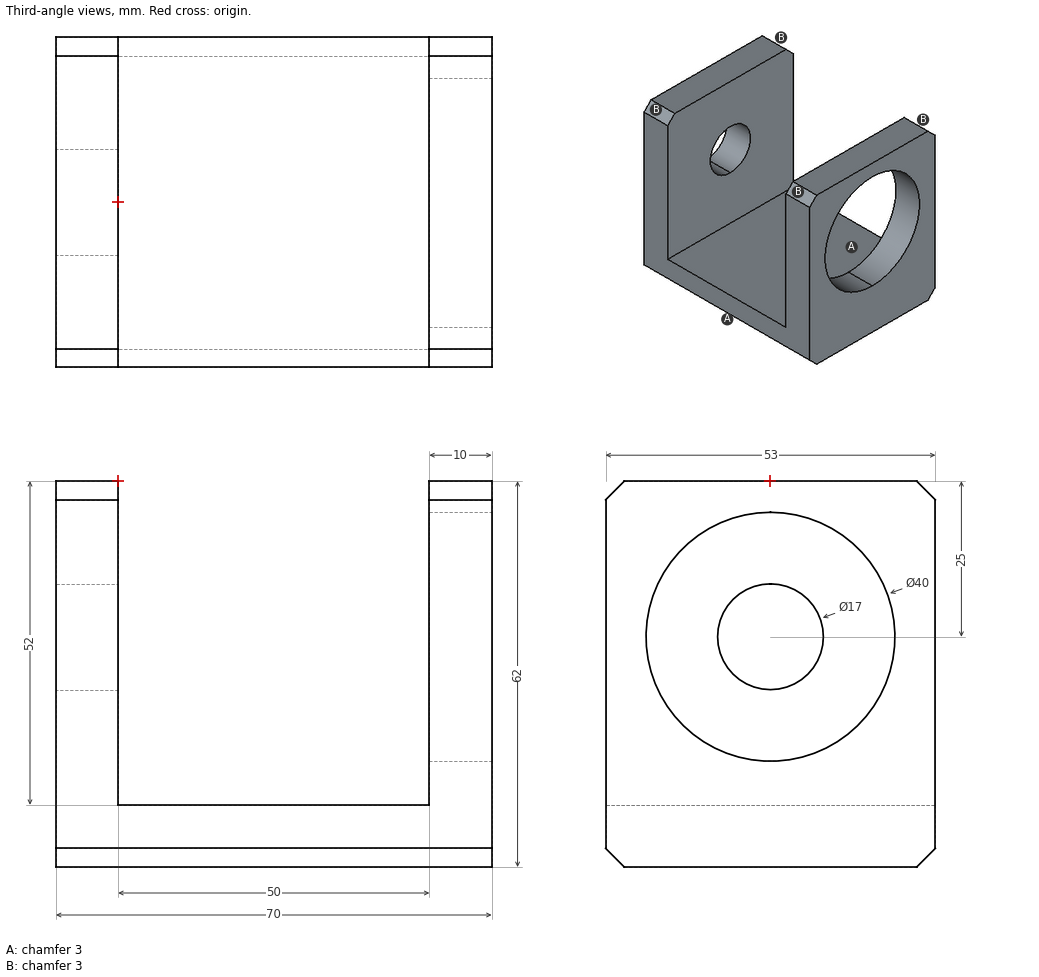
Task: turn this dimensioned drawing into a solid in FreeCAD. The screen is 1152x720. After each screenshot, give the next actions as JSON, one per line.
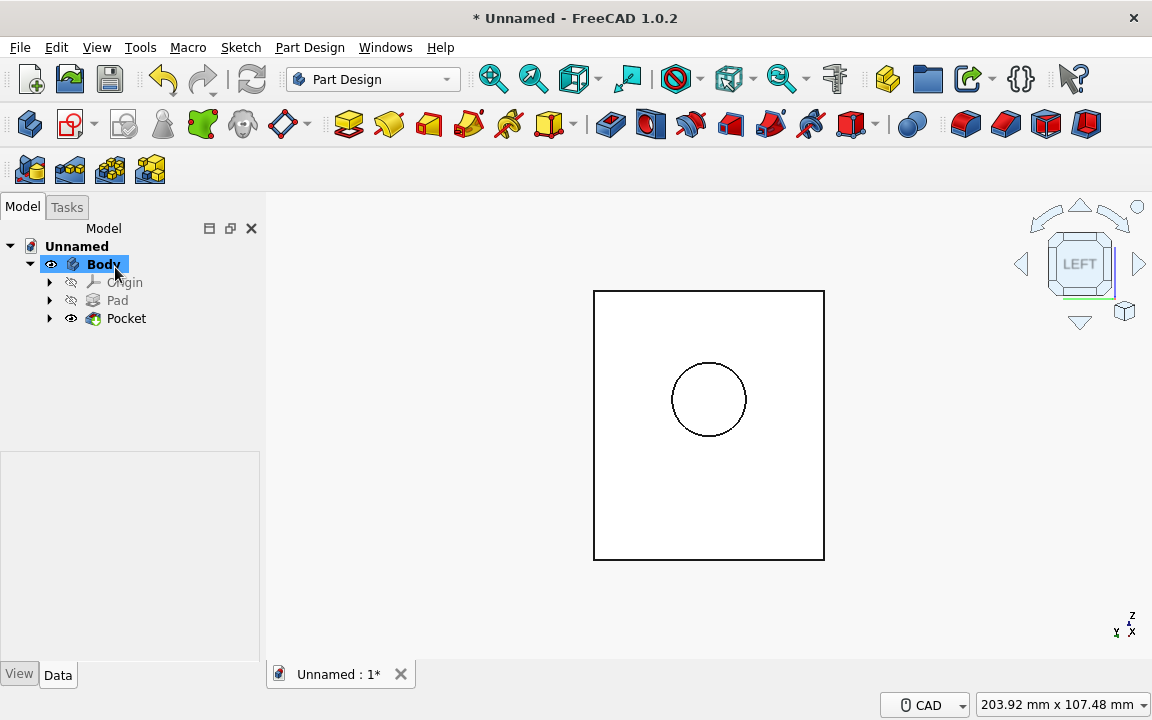
{"action": "left_click", "coordinate": [709, 403]}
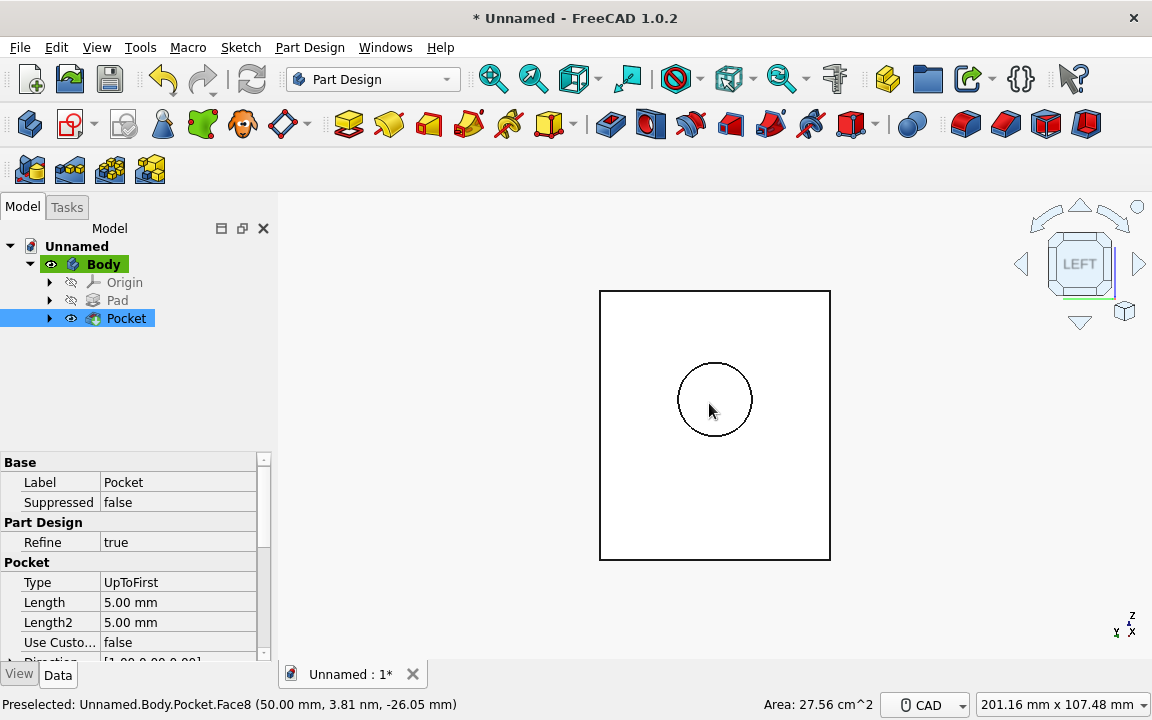
{"action": "left_click", "coordinate": [70, 124]}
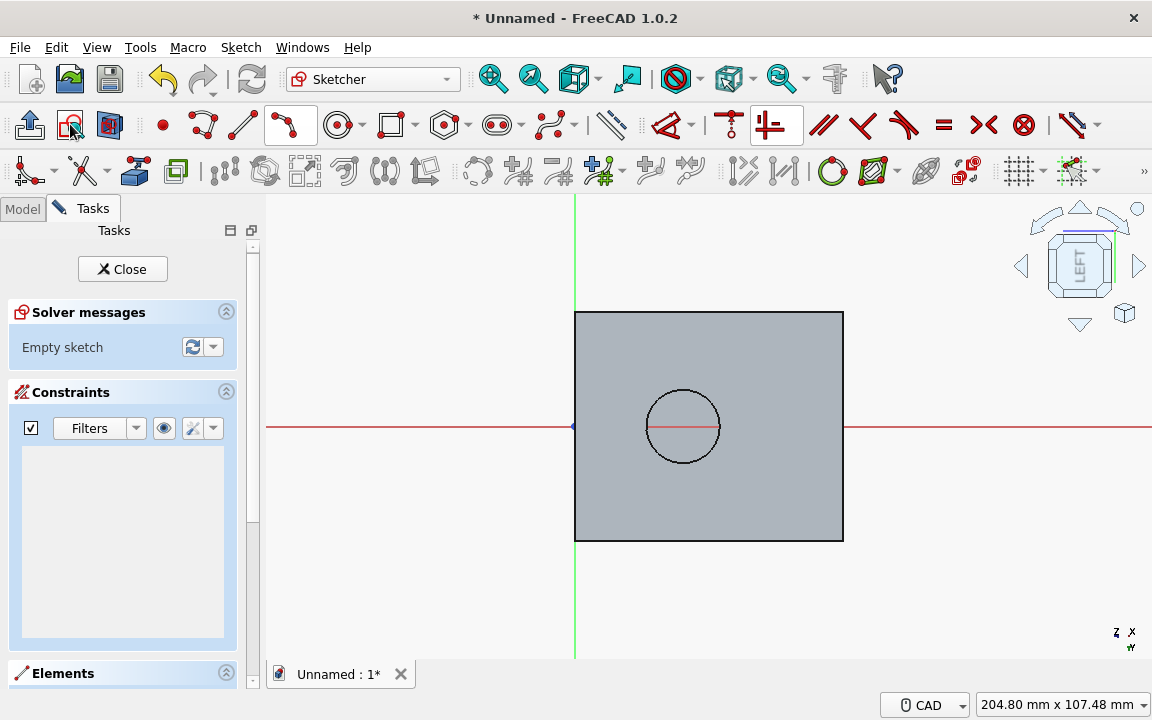
{"action": "left_click", "coordinate": [110, 126]}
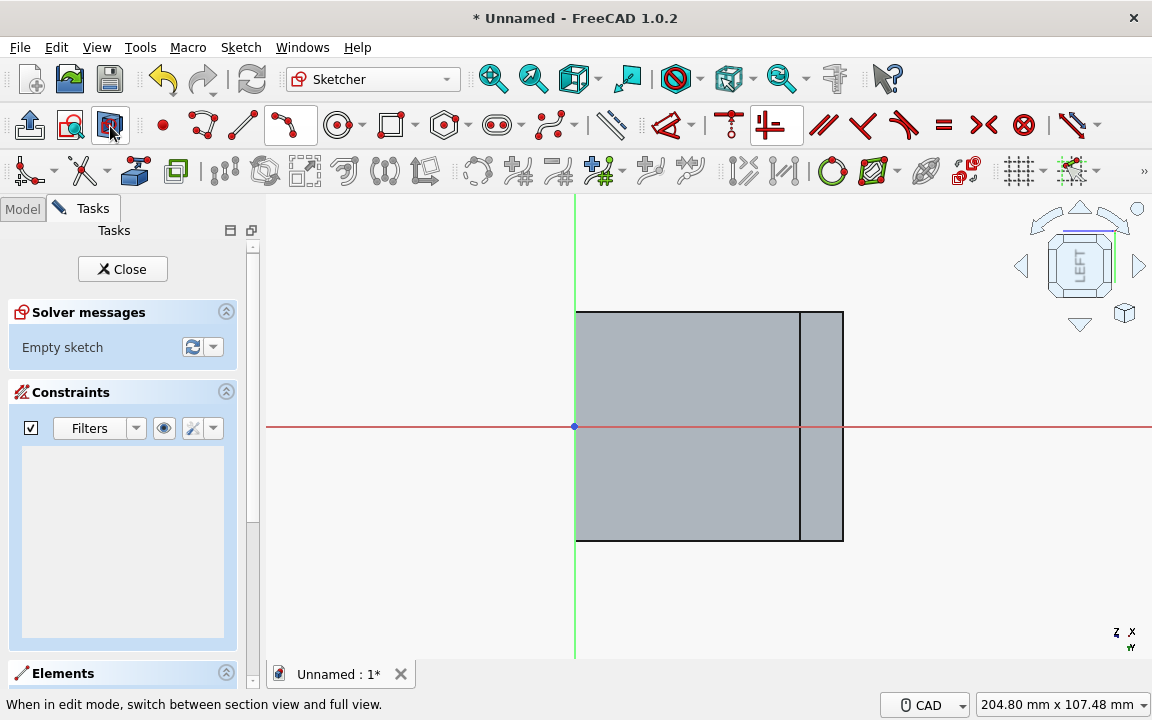
{"action": "scroll", "coordinate": [711, 426], "scroll_direction": "up", "scroll_amount": 3}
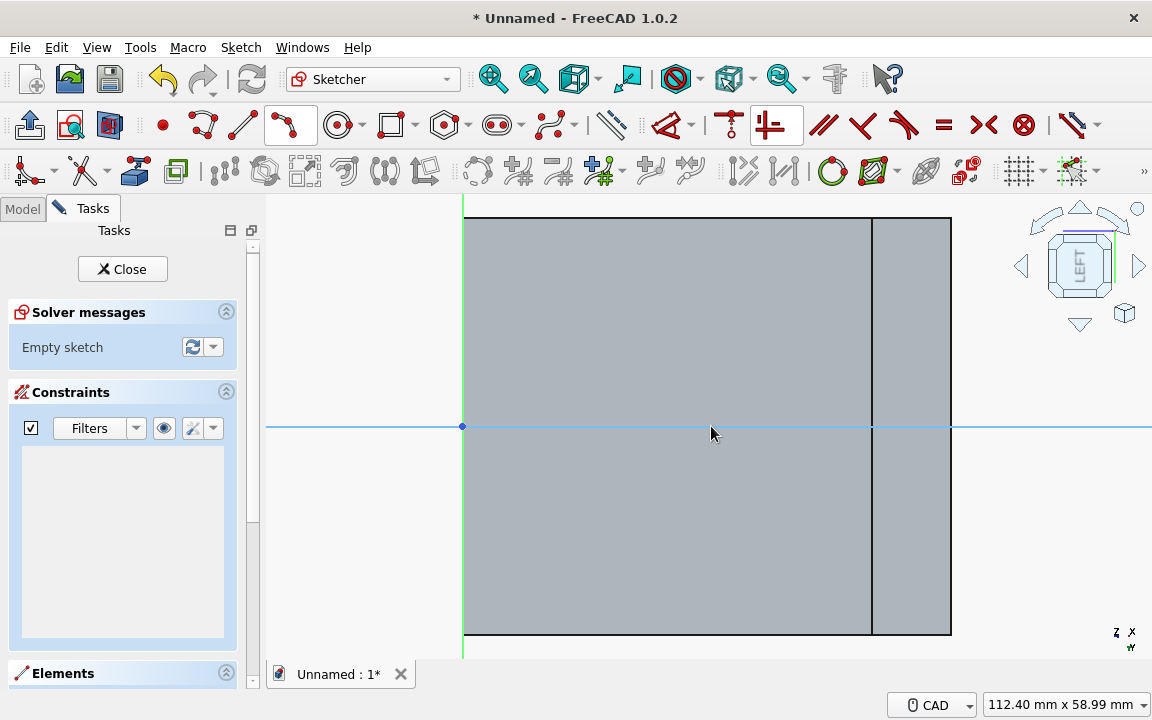
{"action": "key", "text": "g c"}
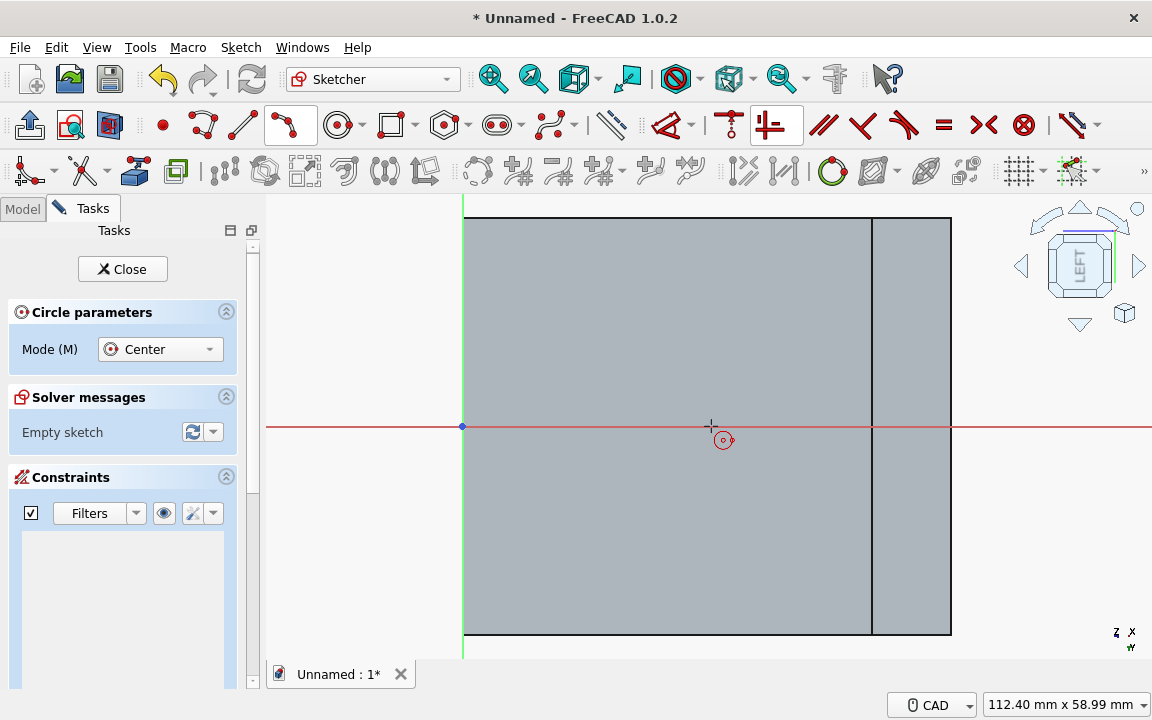
{"action": "left_click", "coordinate": [660, 426]}
{"action": "left_click", "coordinate": [771, 315]}
{"action": "key", "text": "Escape"}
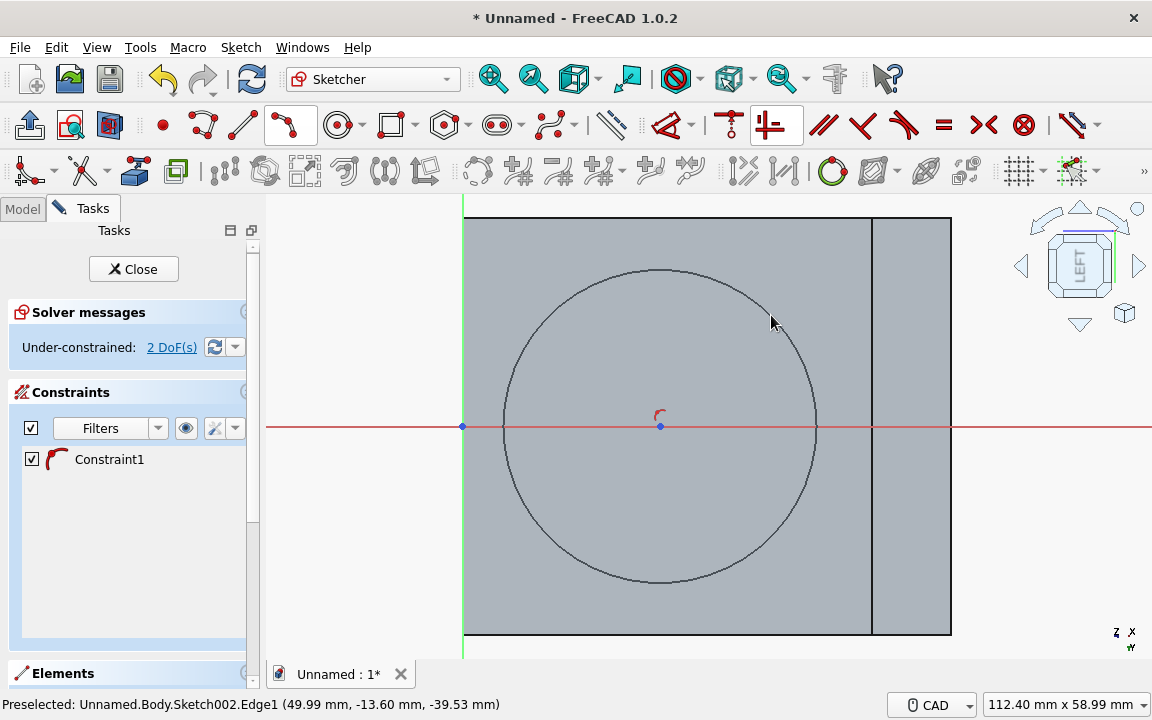
{"action": "key", "text": "d"}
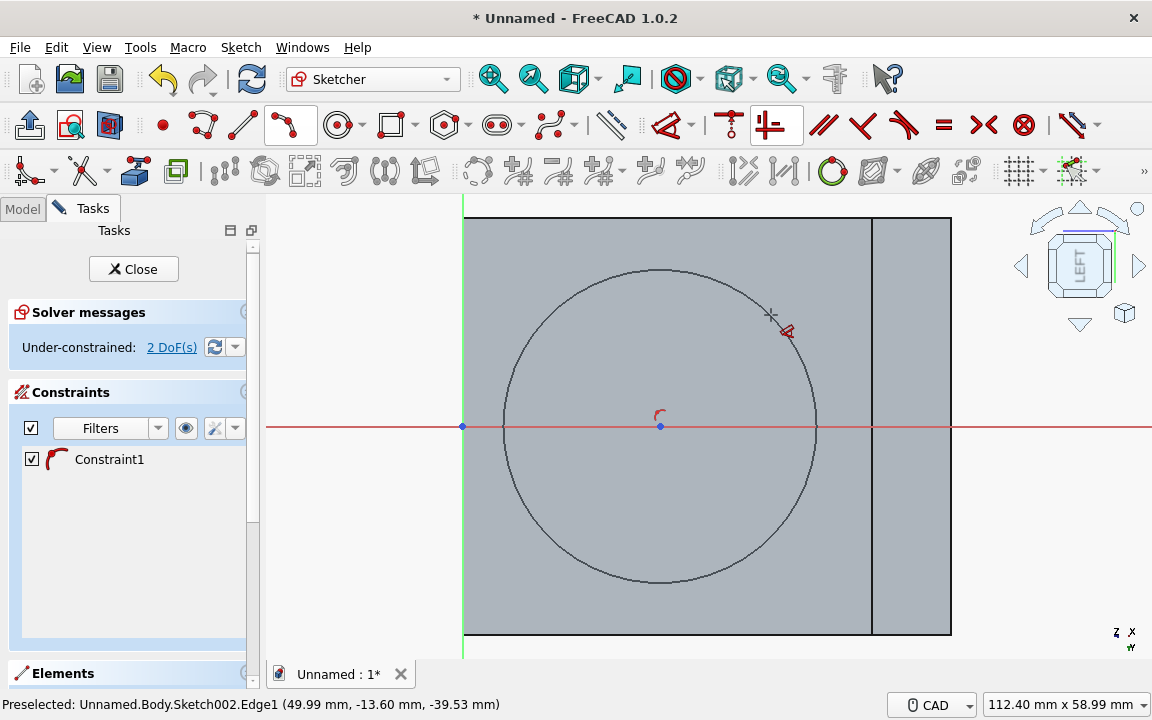
{"action": "left_click", "coordinate": [770, 315]}
{"action": "left_click", "coordinate": [792, 292]}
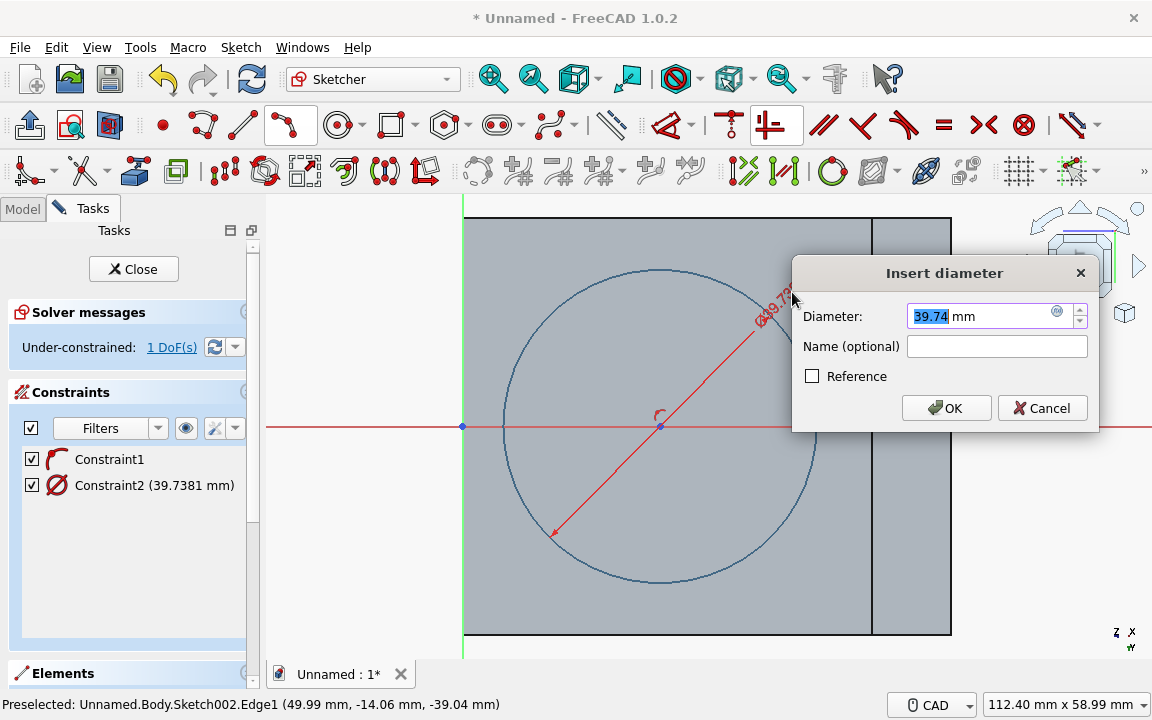
{"action": "type", "text": "40"}
{"action": "key", "text": "Return"}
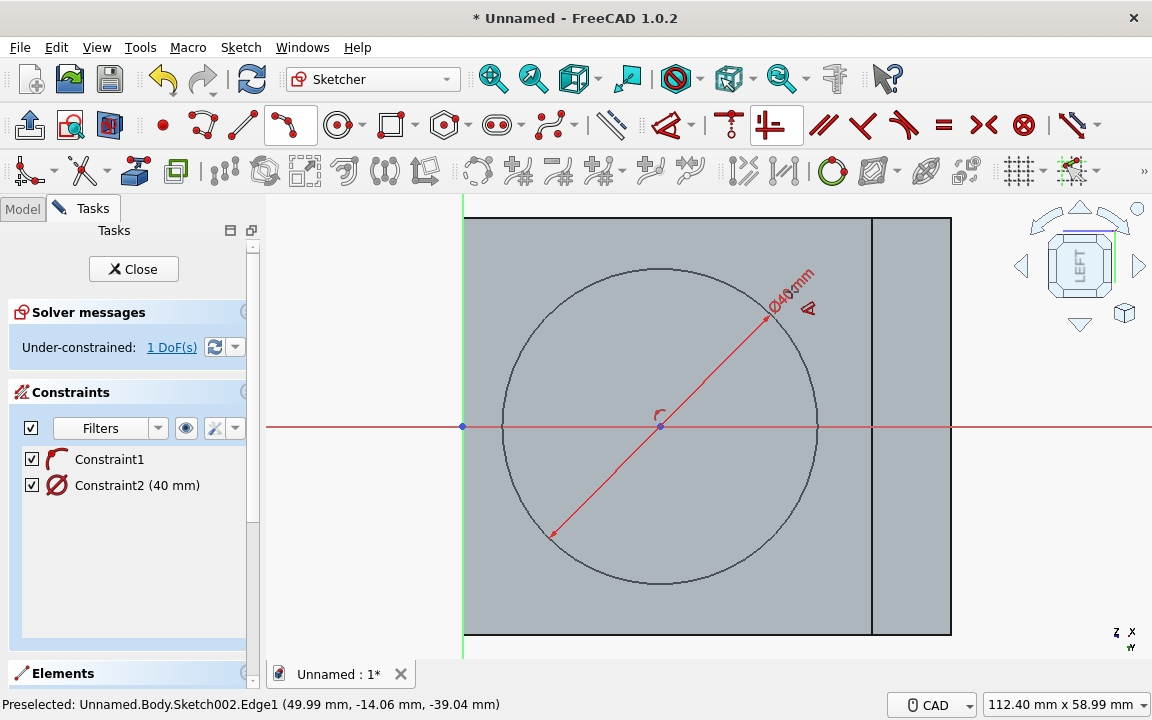
{"action": "left_click", "coordinate": [660, 426]}
{"action": "left_click", "coordinate": [561, 460]}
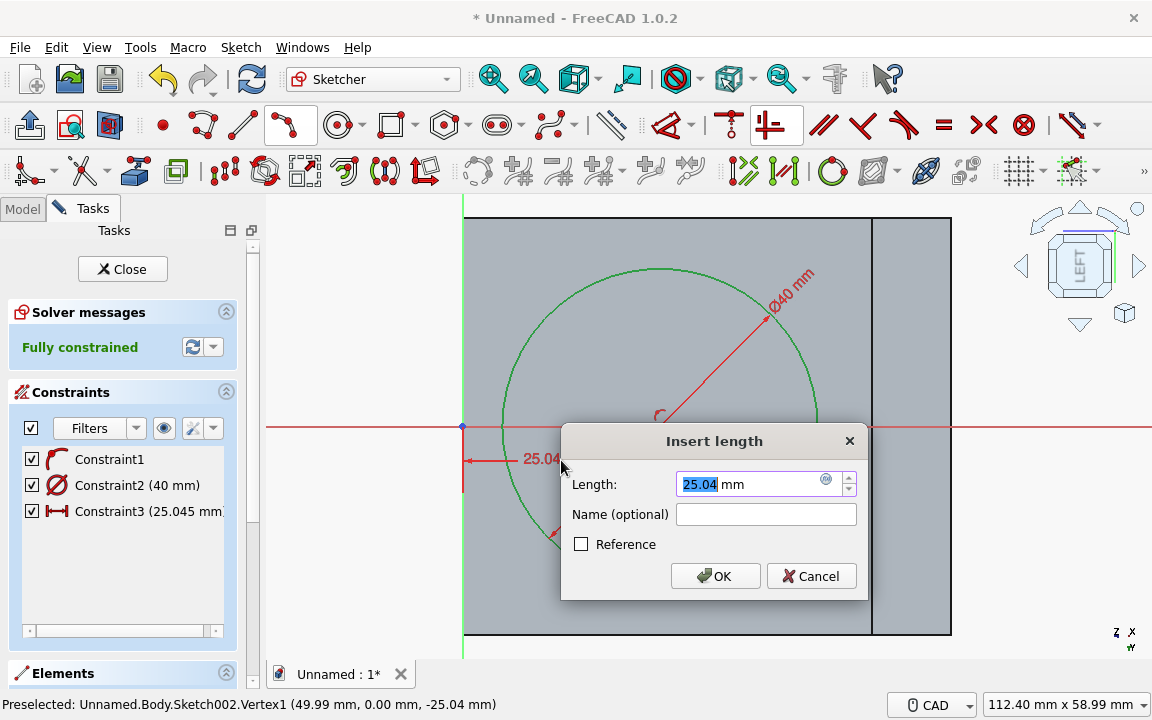
{"action": "type", "text": "25"}
{"action": "key", "text": "Return"}
{"action": "key", "text": "Escape"}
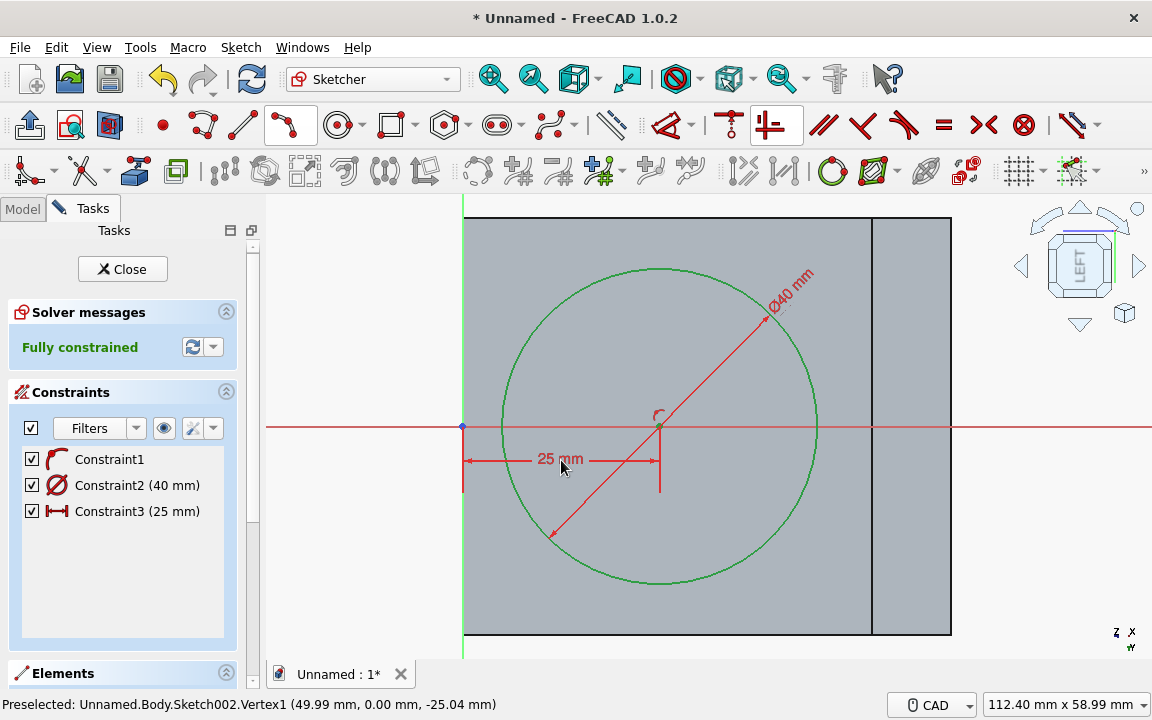
{"action": "left_click", "coordinate": [123, 269]}